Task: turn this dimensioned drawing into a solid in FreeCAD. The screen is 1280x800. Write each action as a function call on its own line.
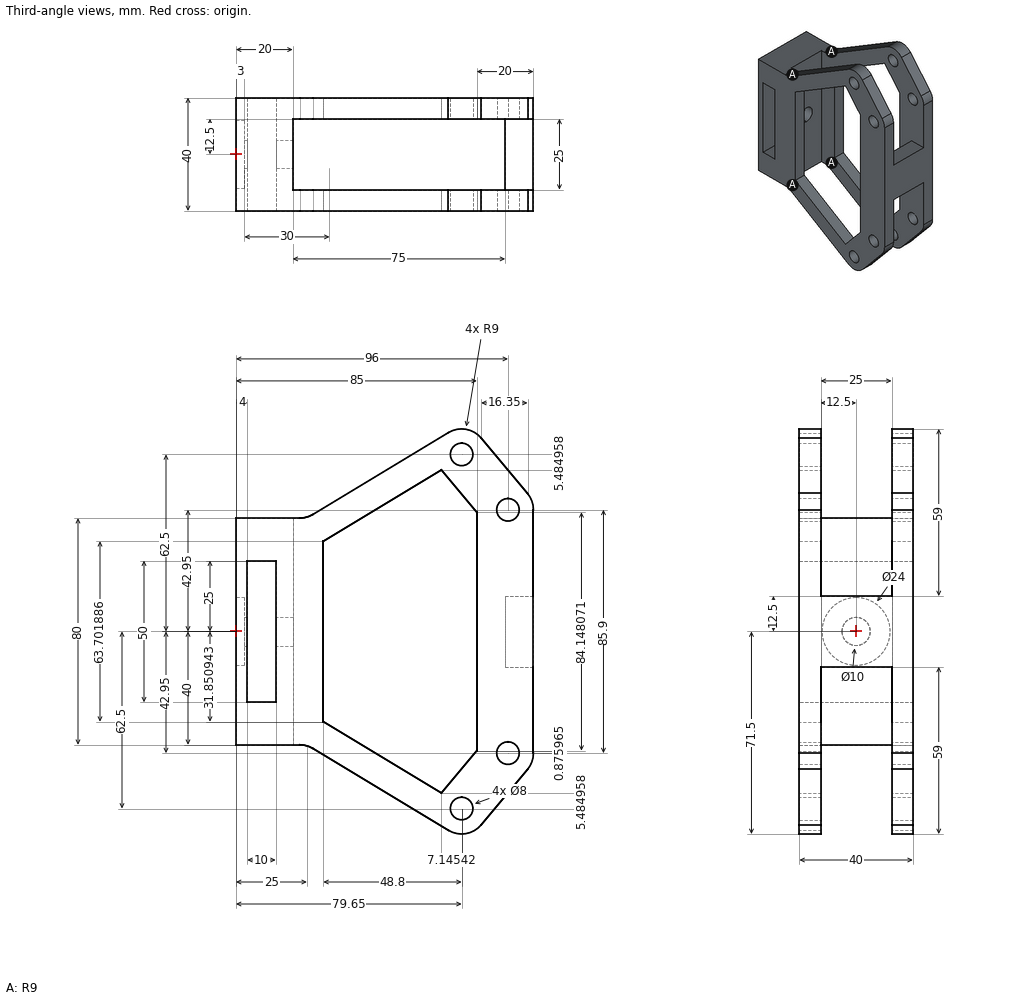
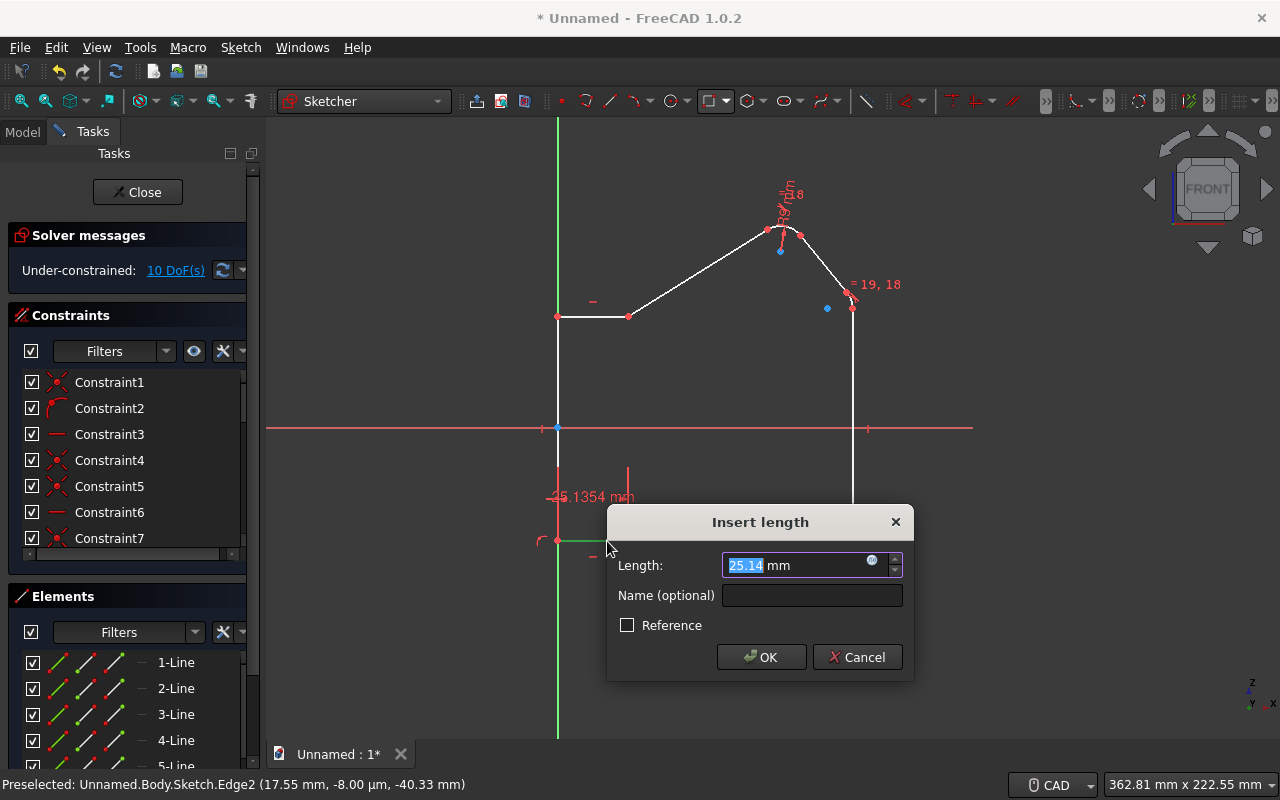
text(25)
key(Return)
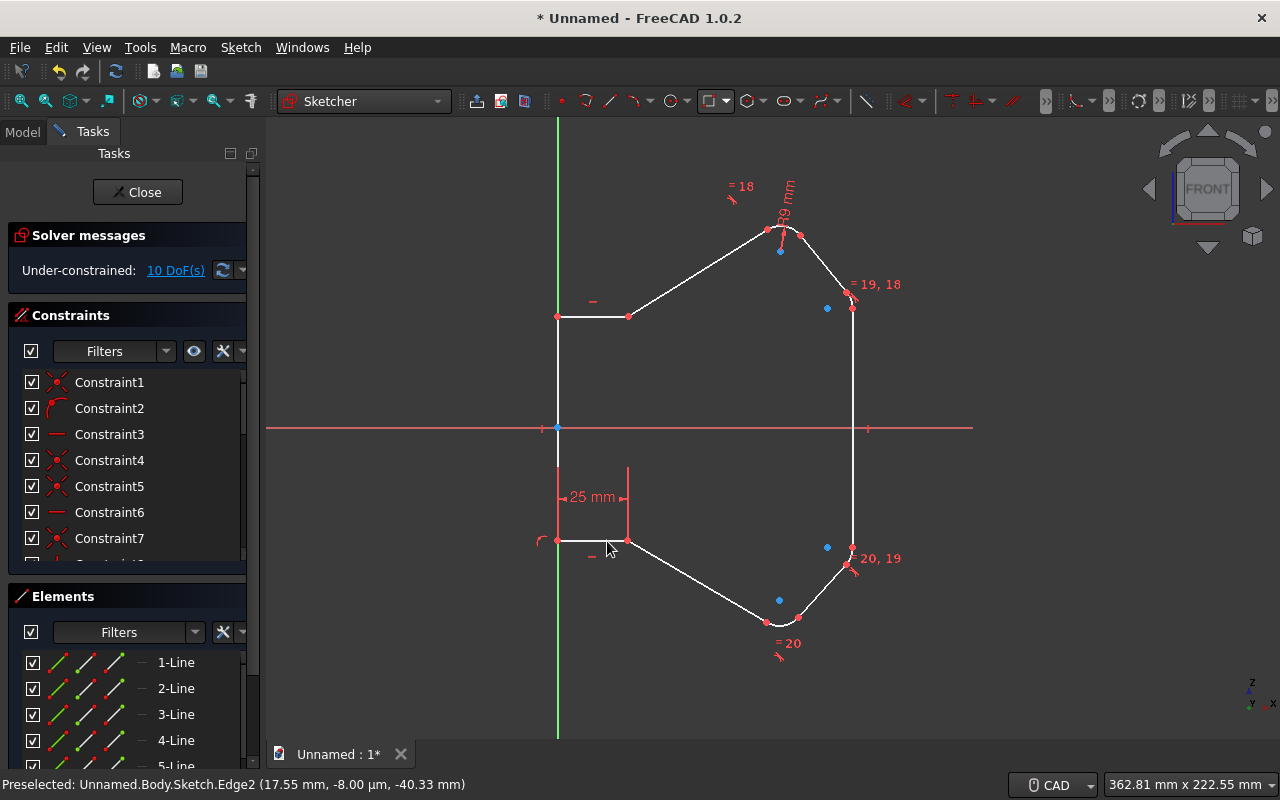
click(558, 473)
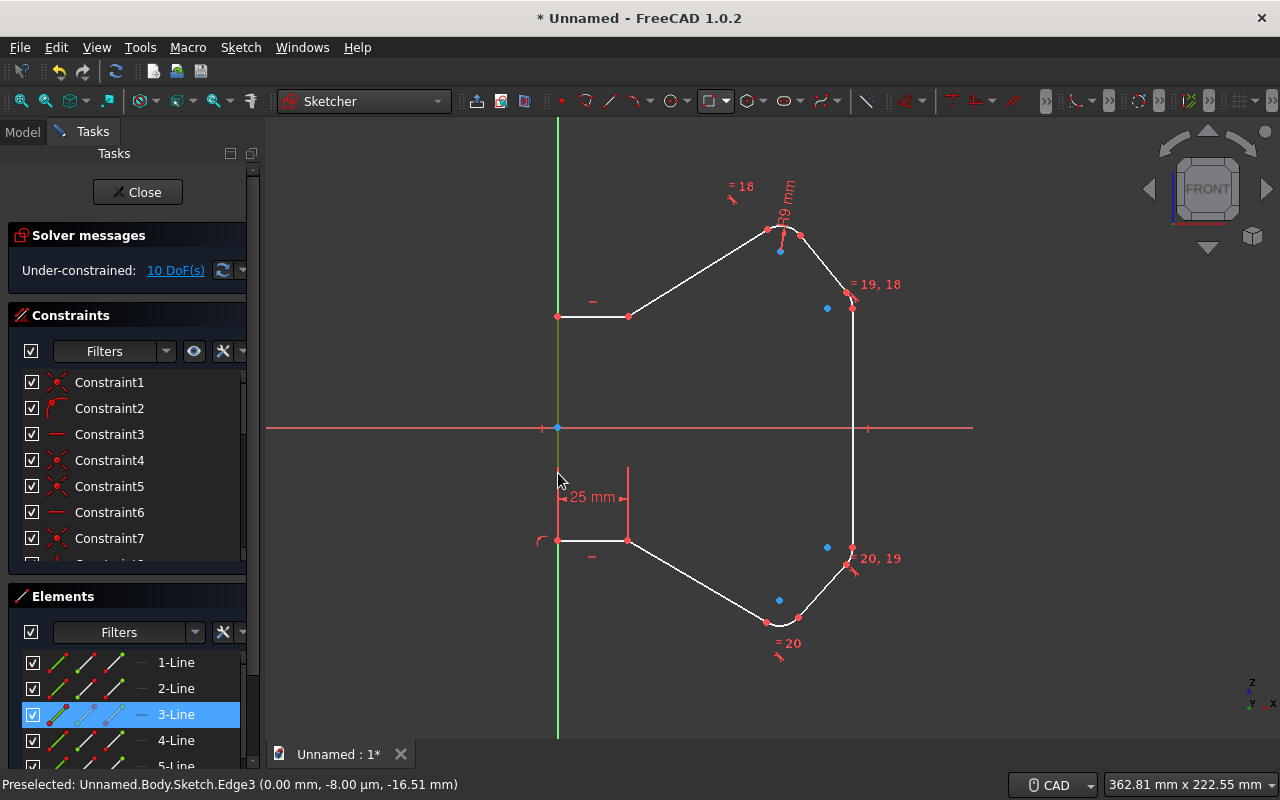
key(i)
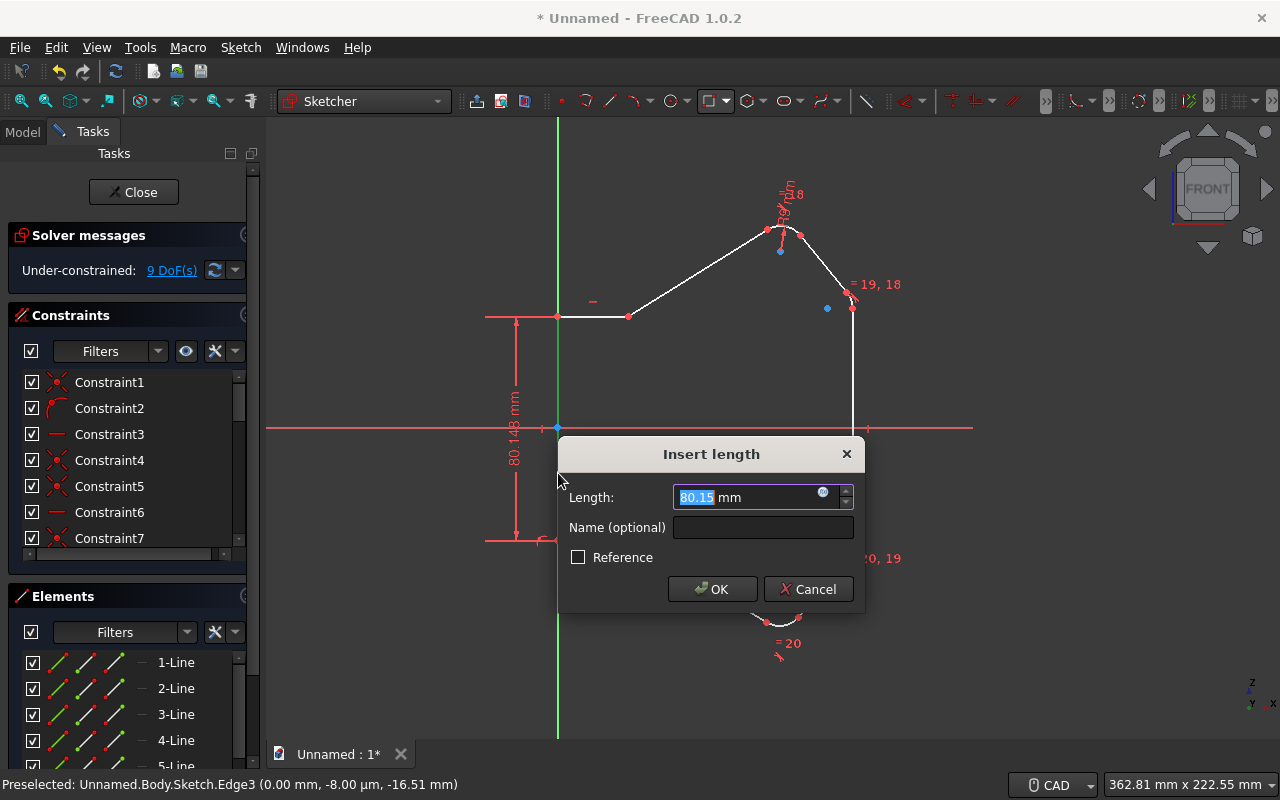
text(80)
key(Return)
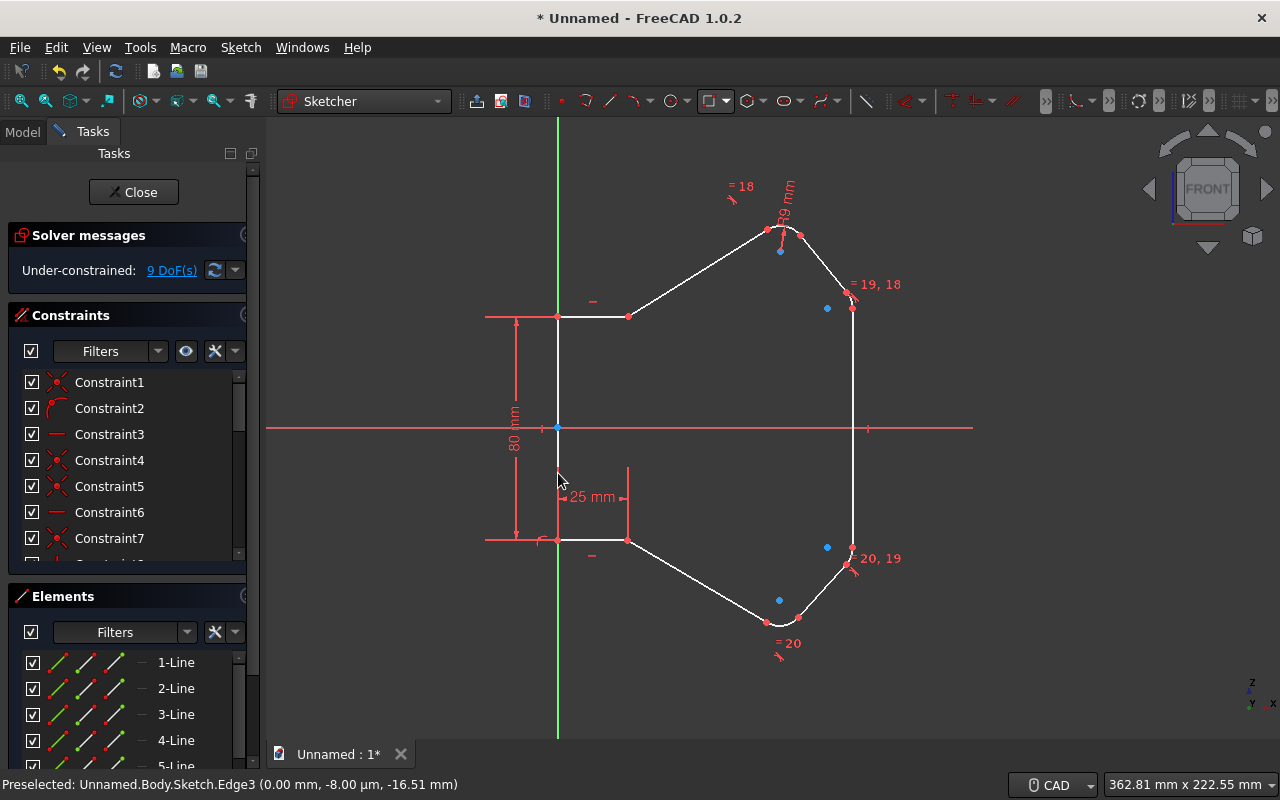
click(579, 317)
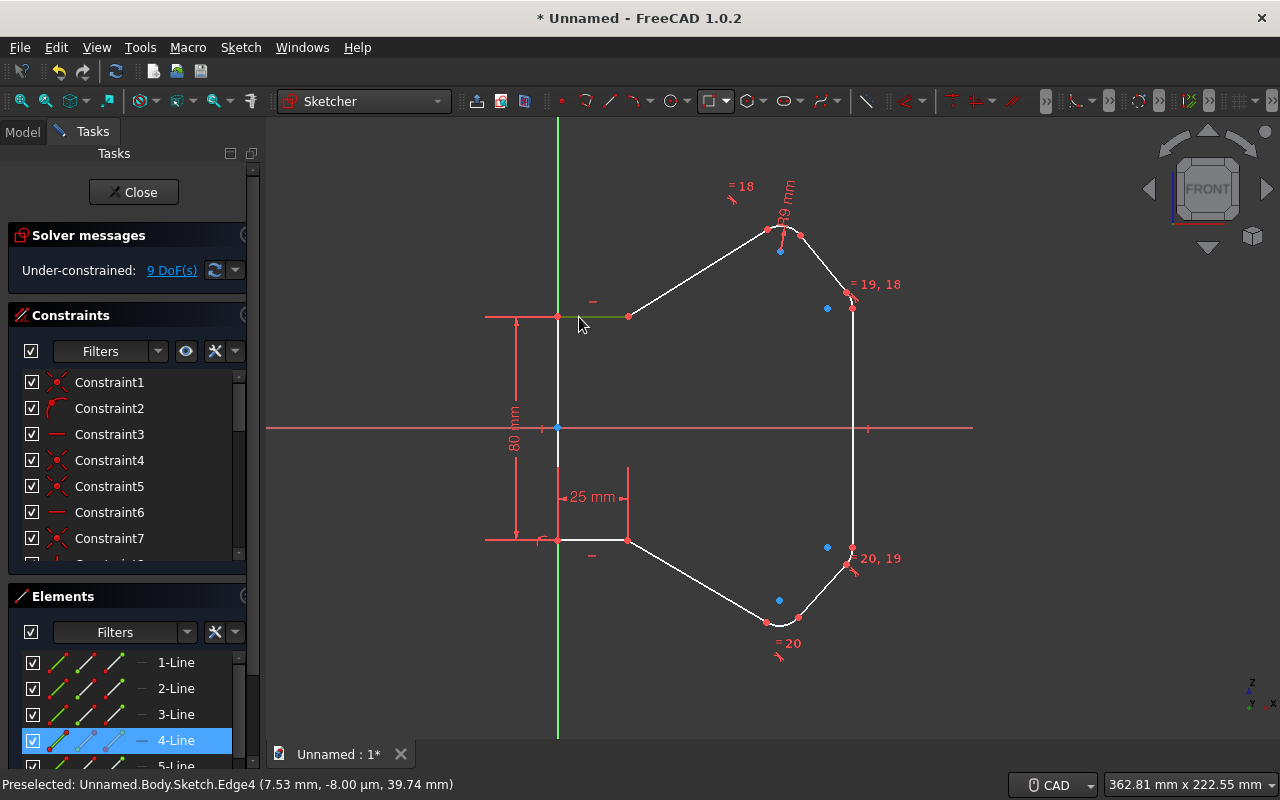
click(924, 102)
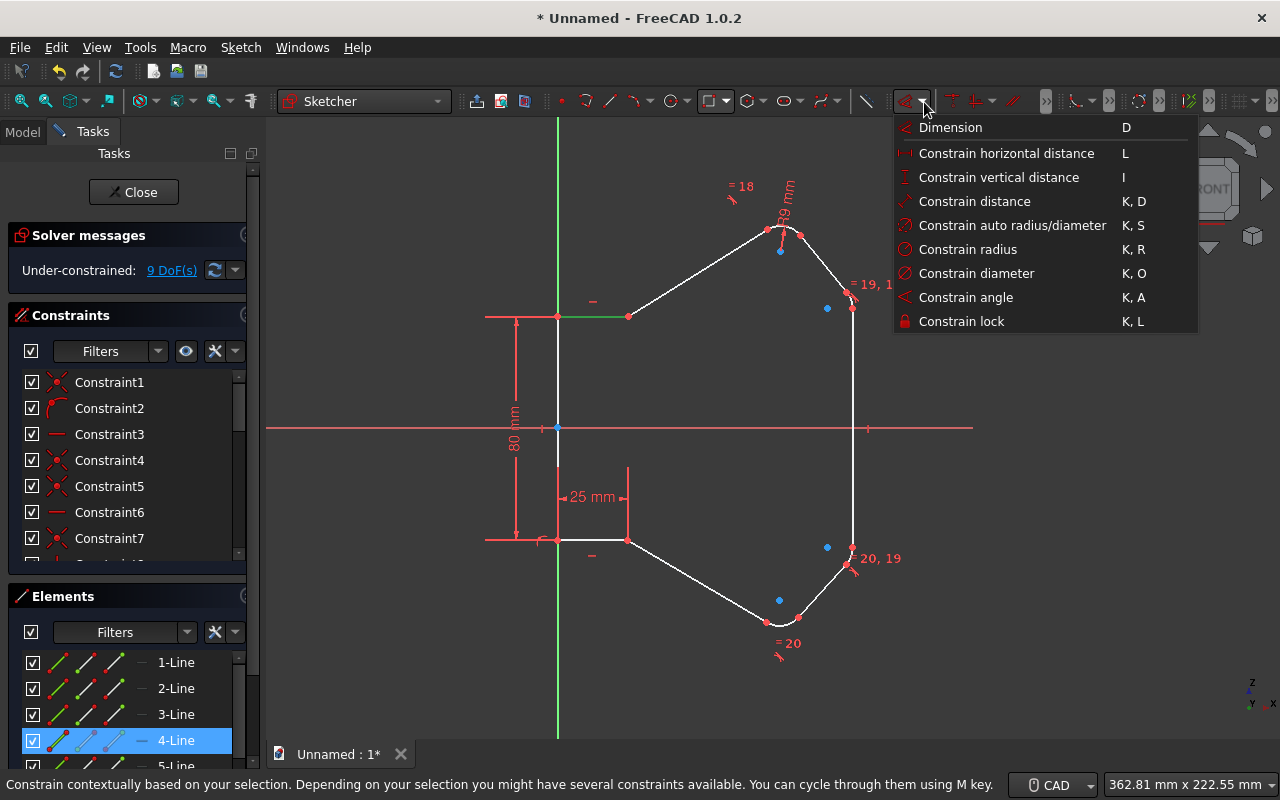
click(1046, 153)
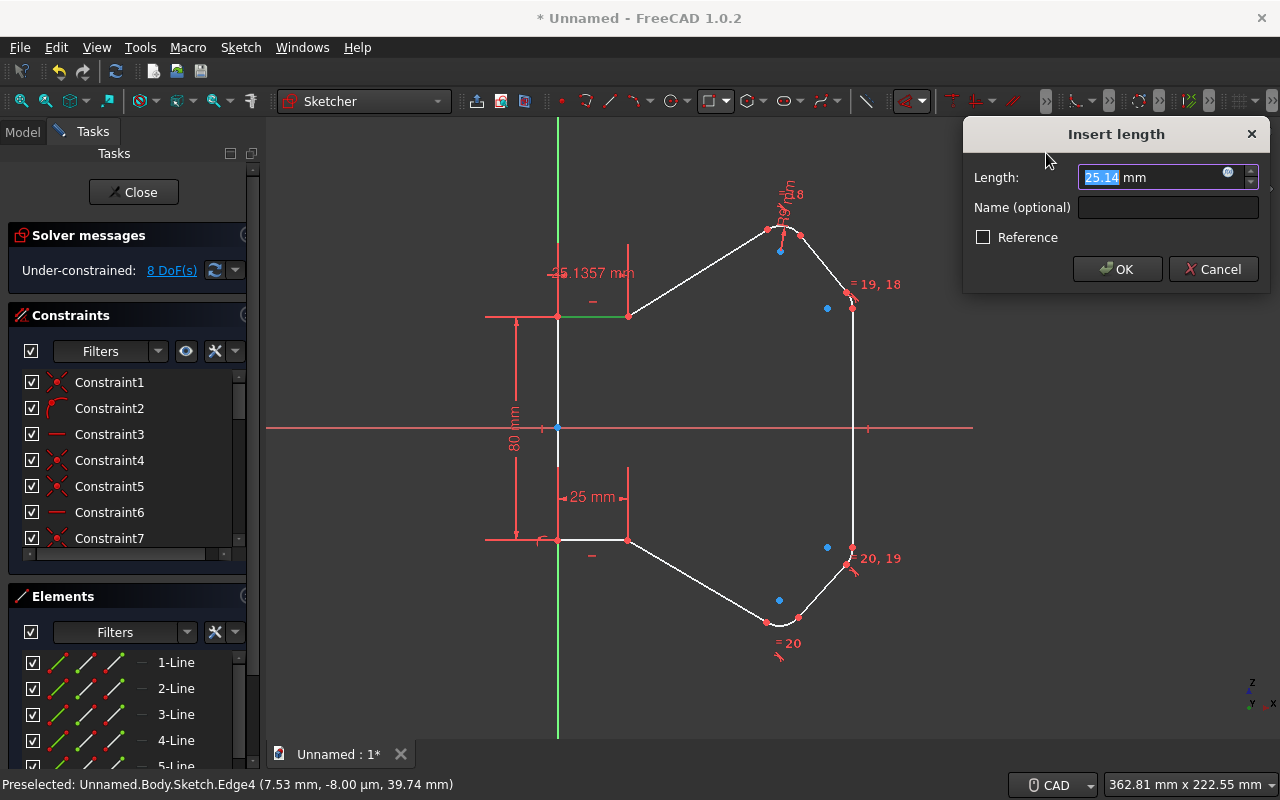
text(25)
key(Return)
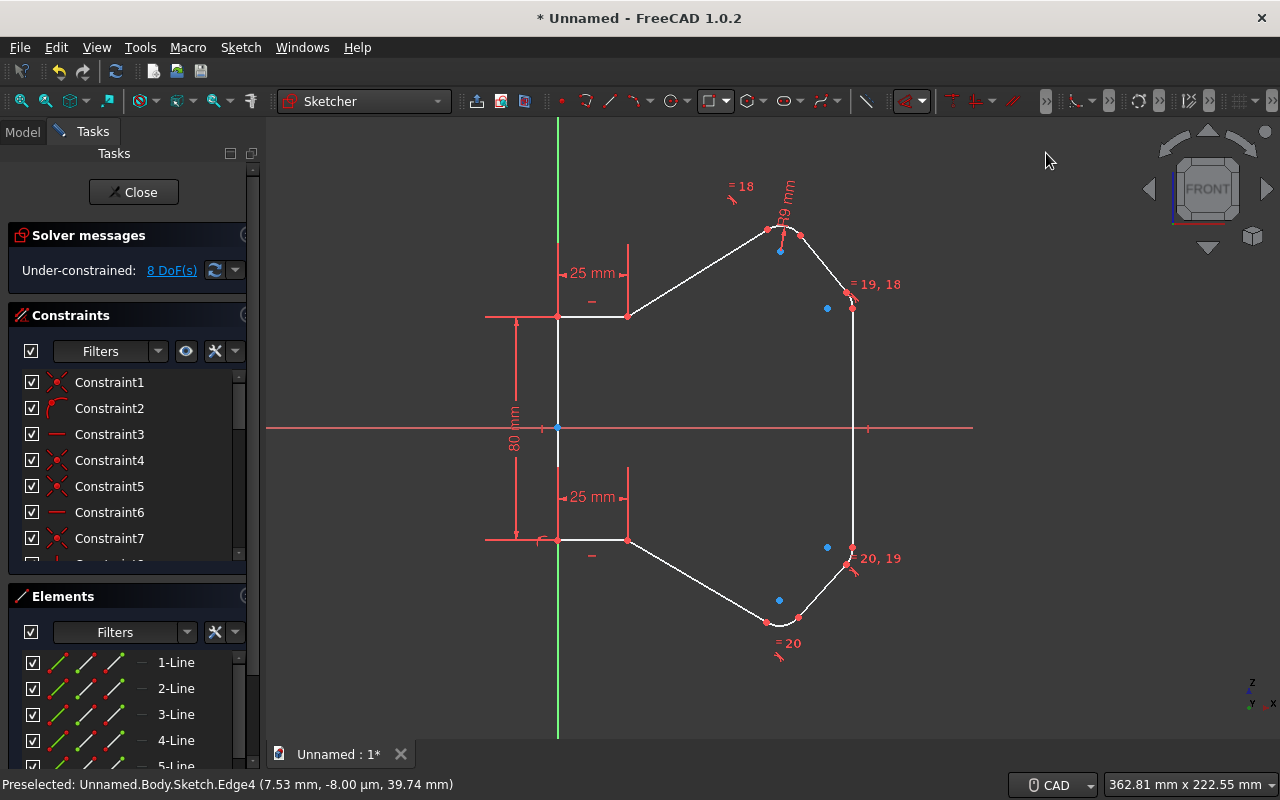
click(628, 540)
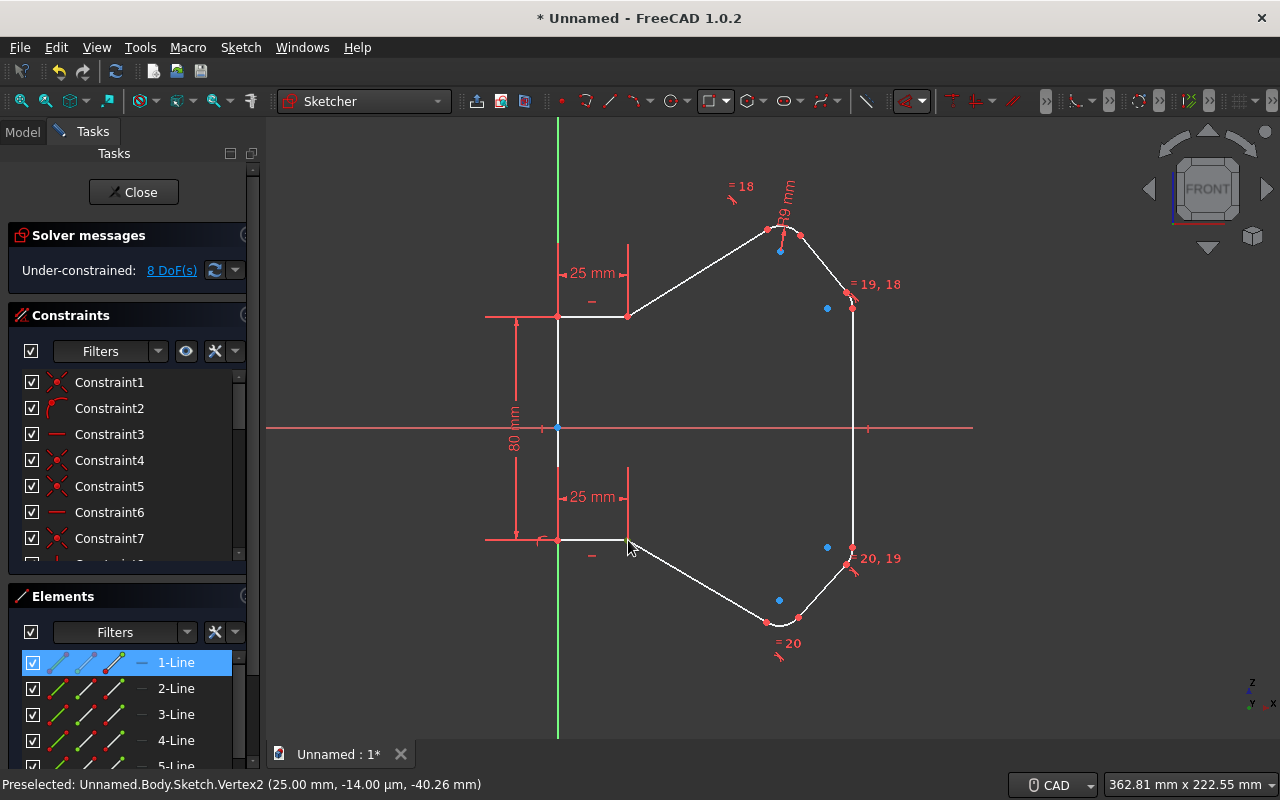
key(i)